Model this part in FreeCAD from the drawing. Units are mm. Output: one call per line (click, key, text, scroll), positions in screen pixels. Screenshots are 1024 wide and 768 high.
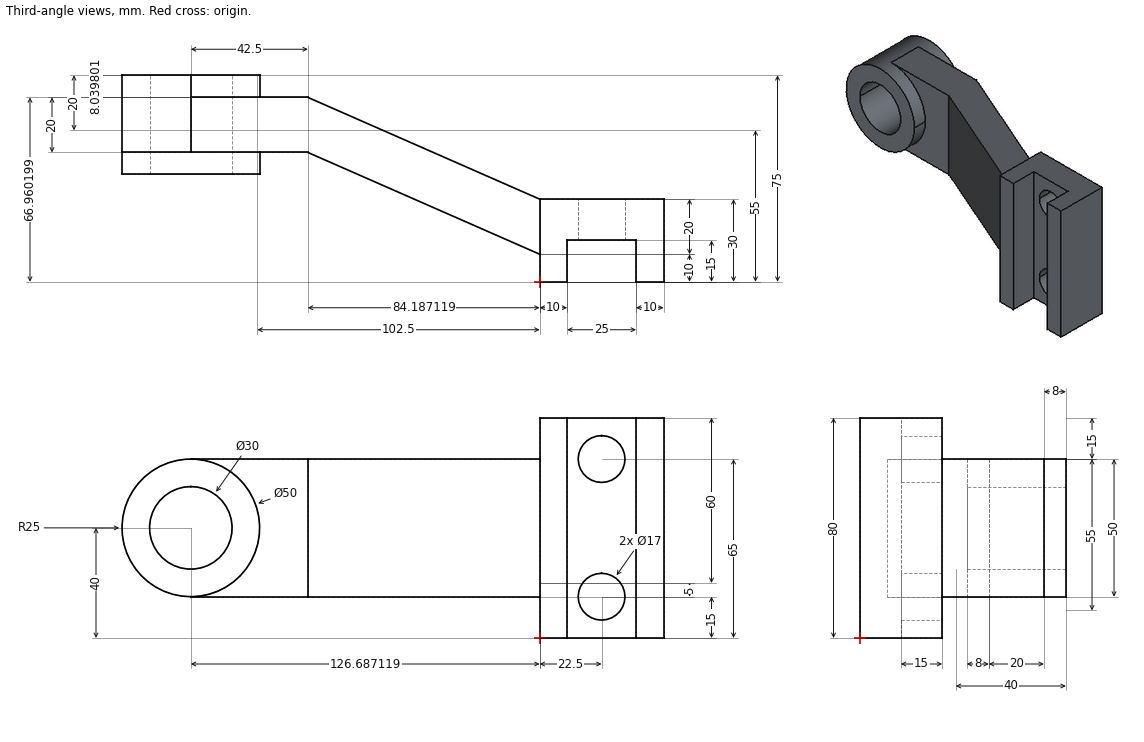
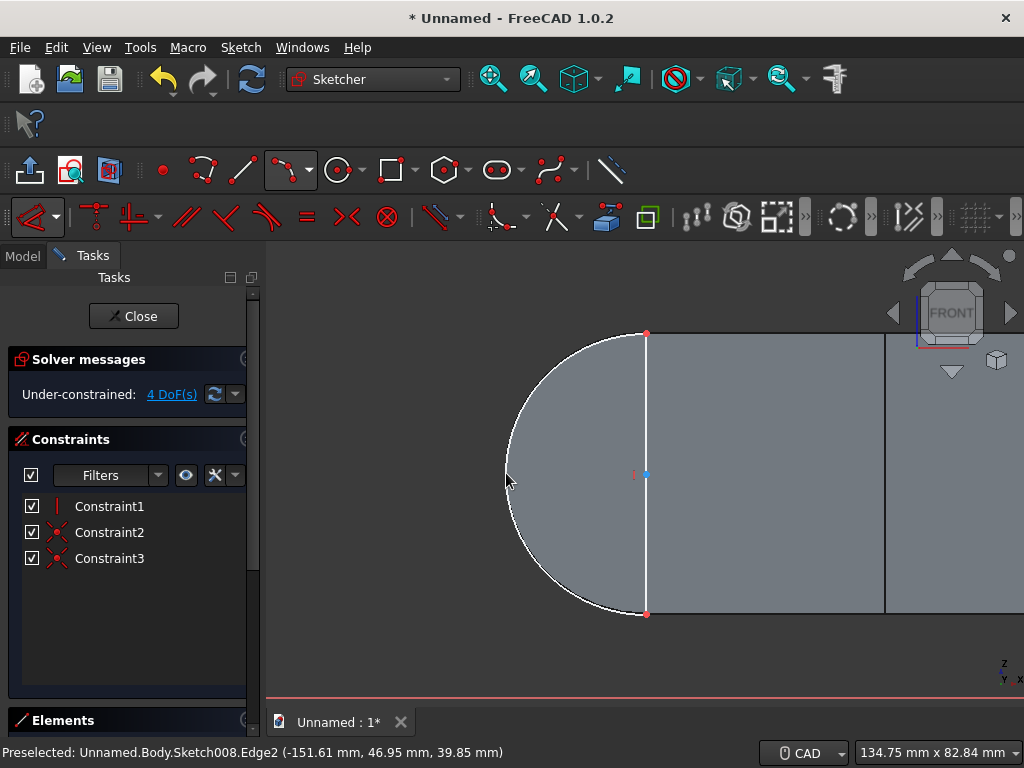
click(533, 392)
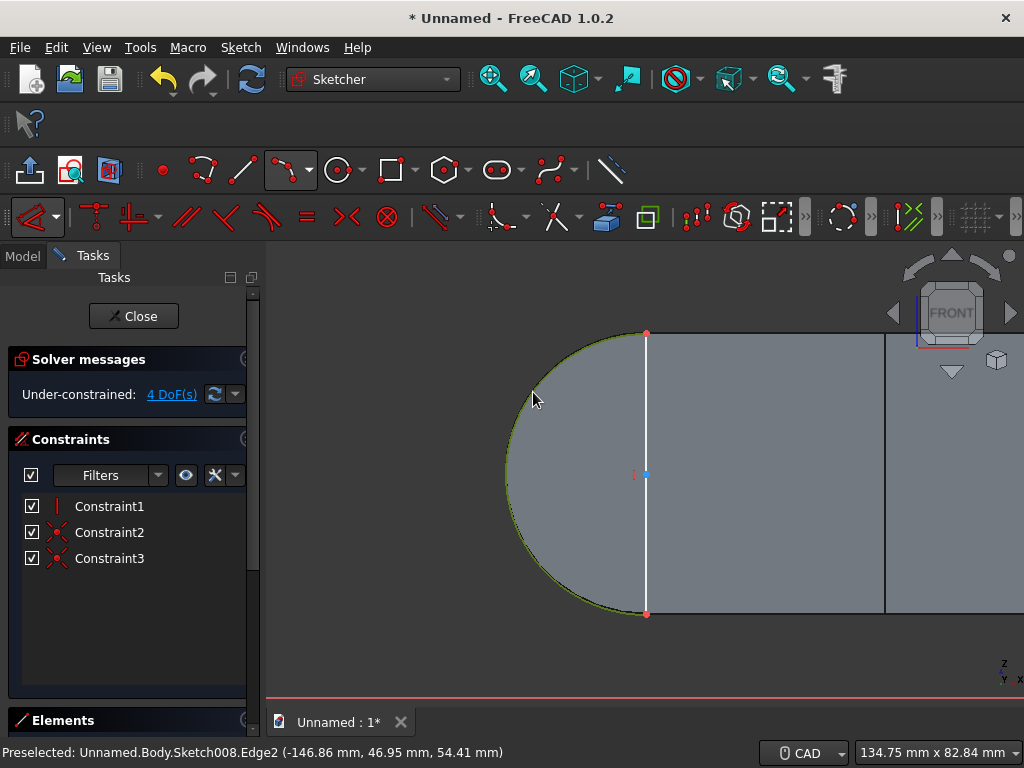
key(k)
key(r)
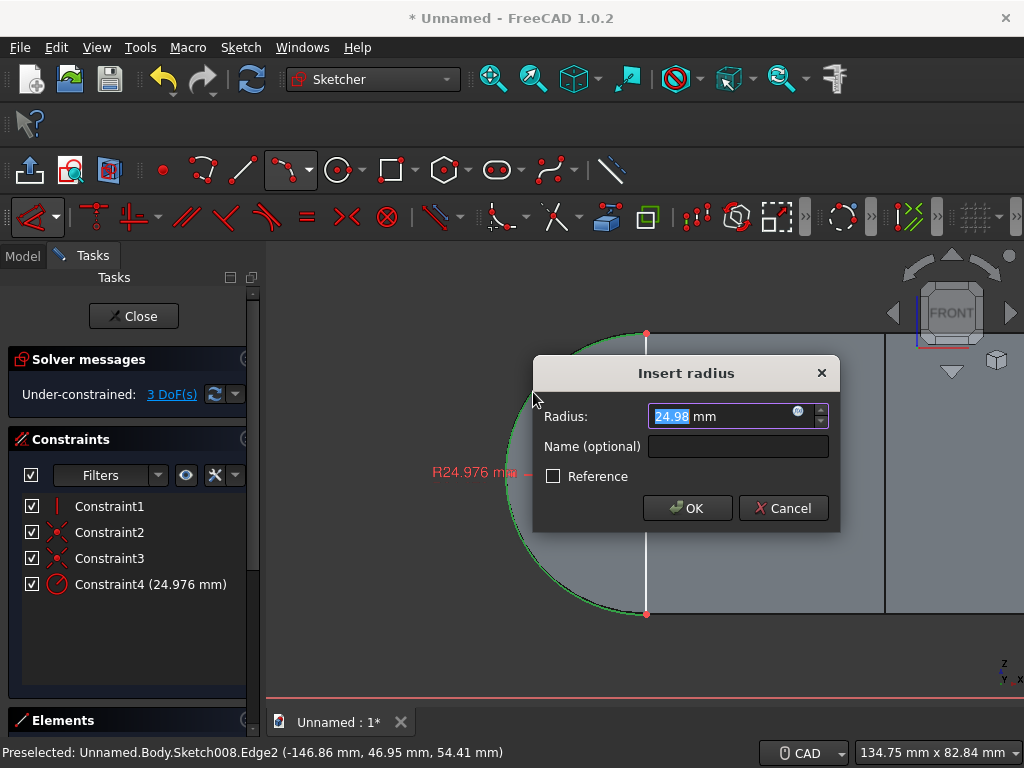
text(25)
key(Return)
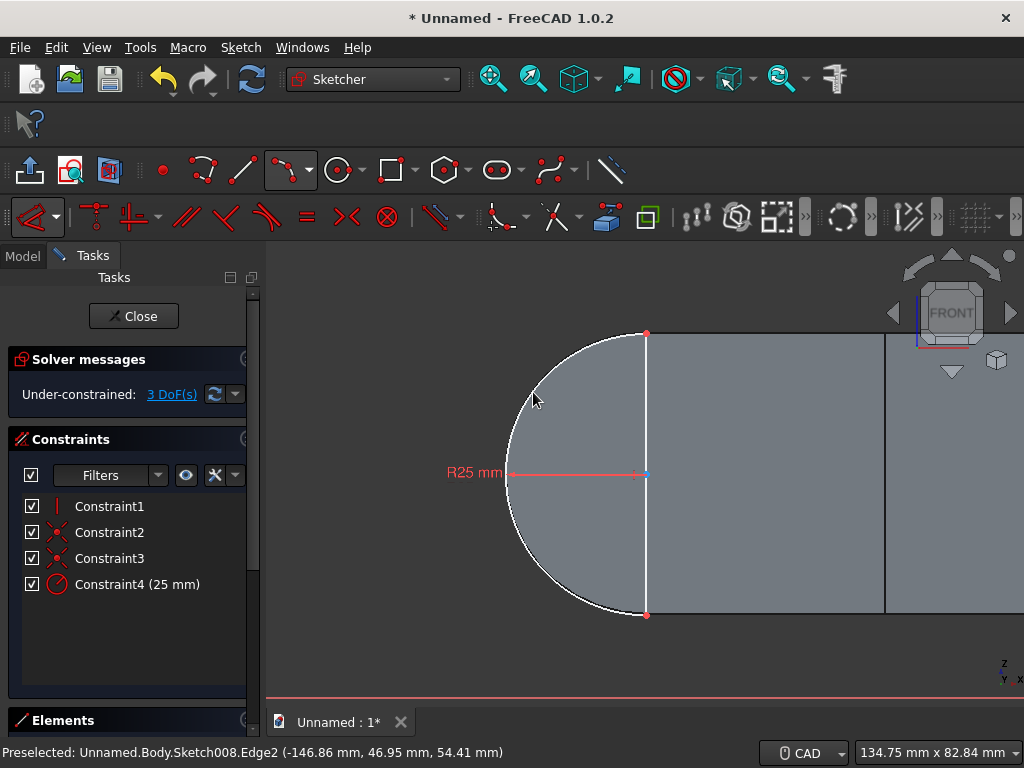
click(646, 615)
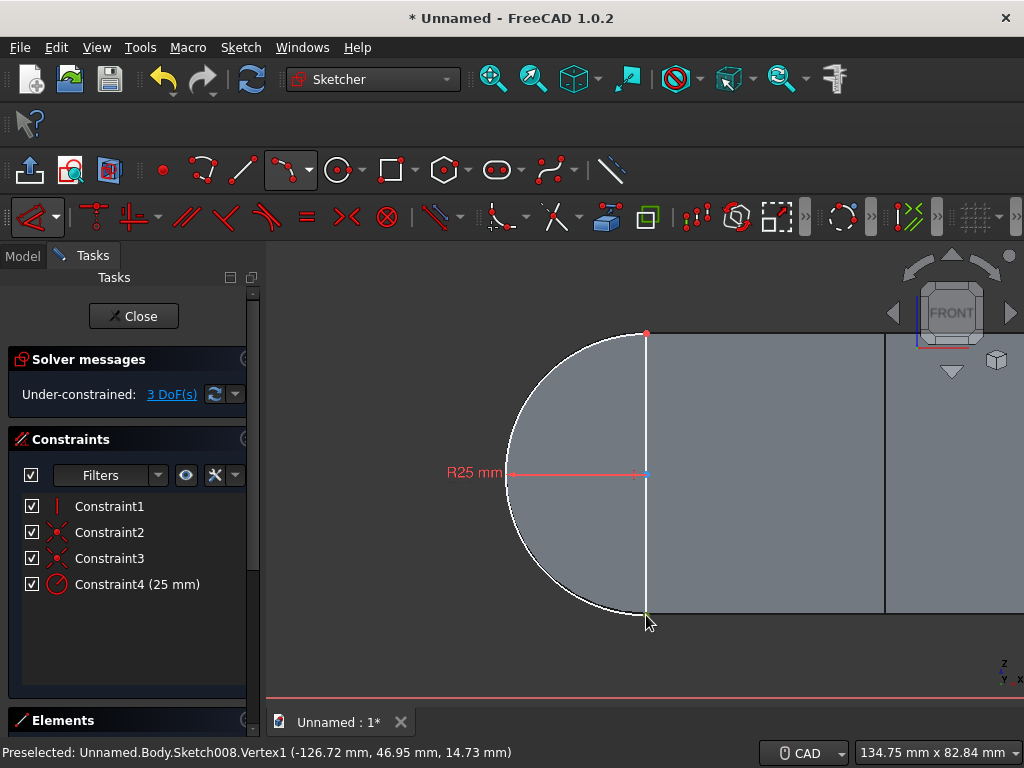
key(i)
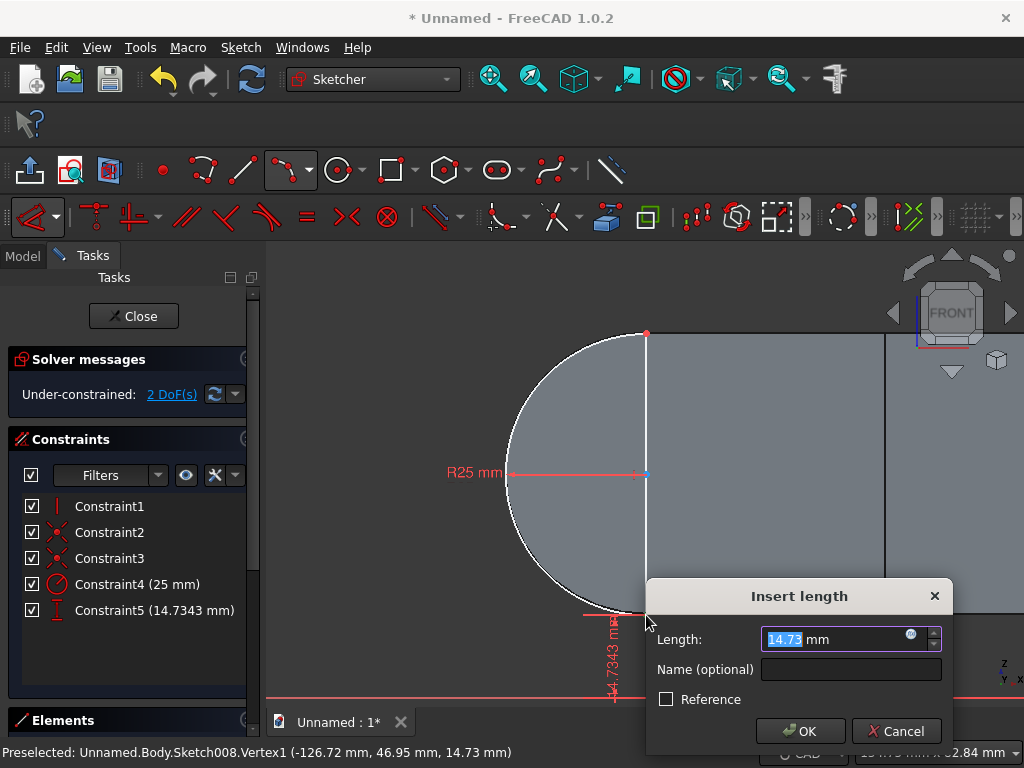
text(15)
key(Return)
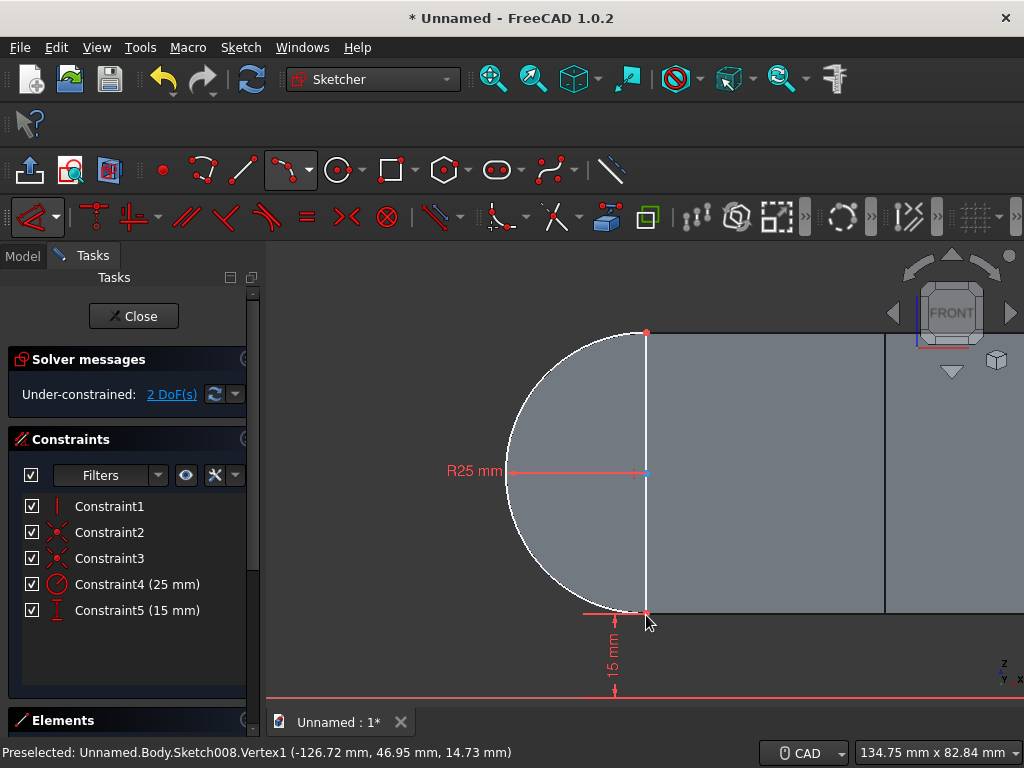
click(646, 614)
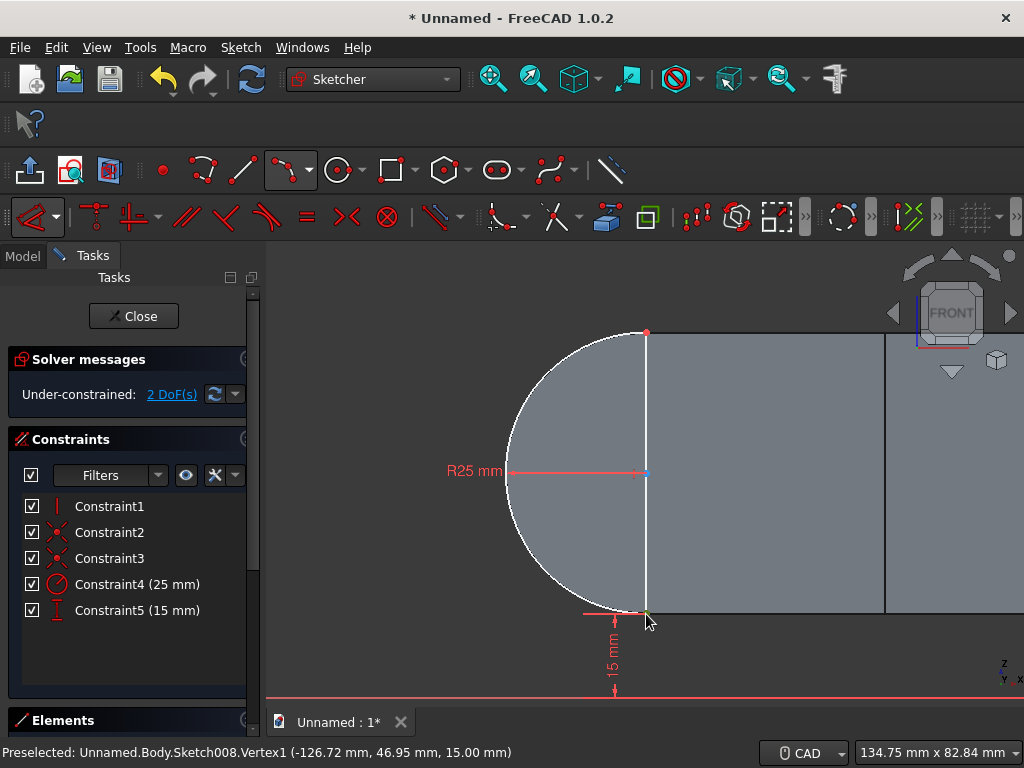
key(l)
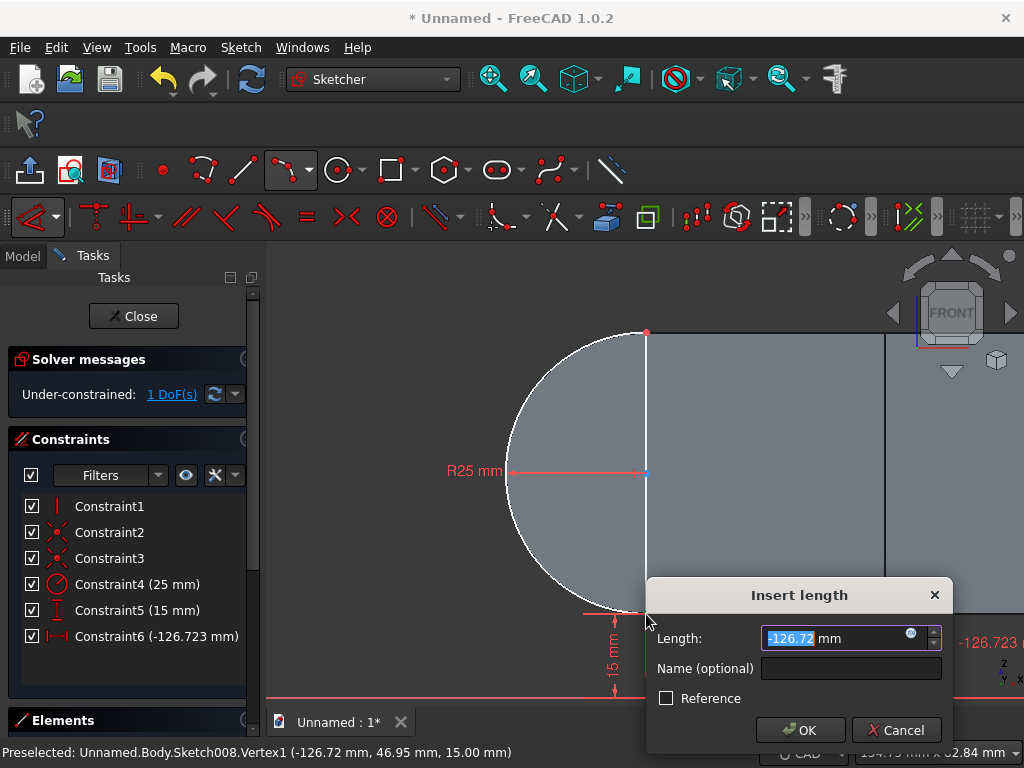
text(-126.687119)
key(Return)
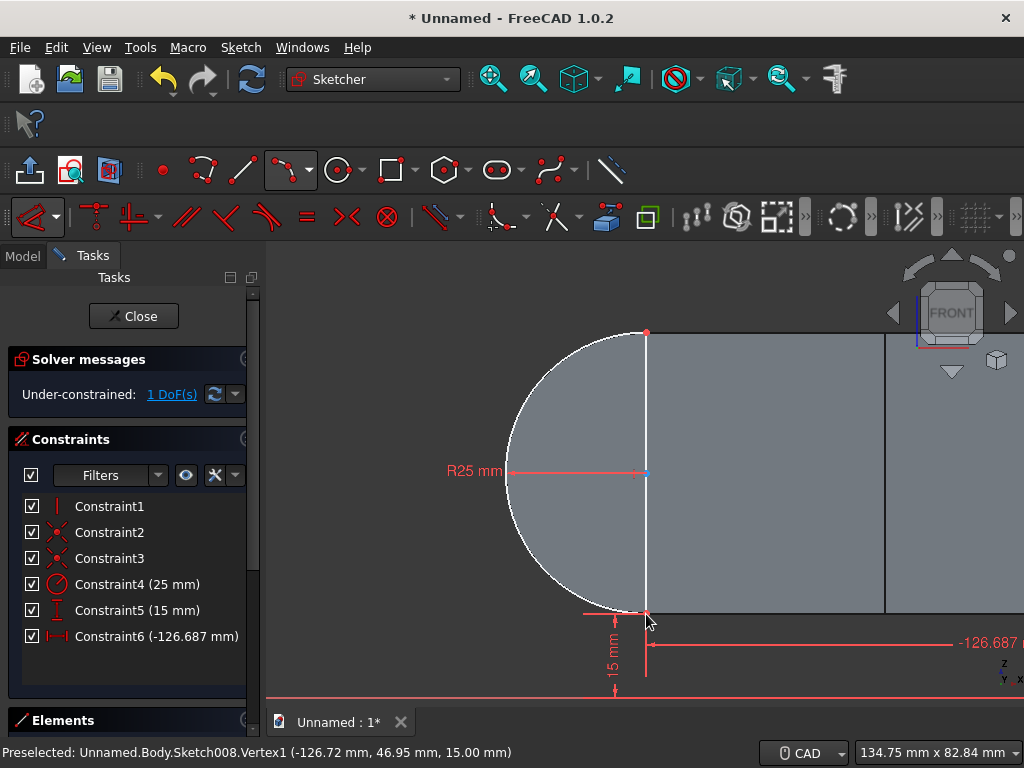
click(647, 473)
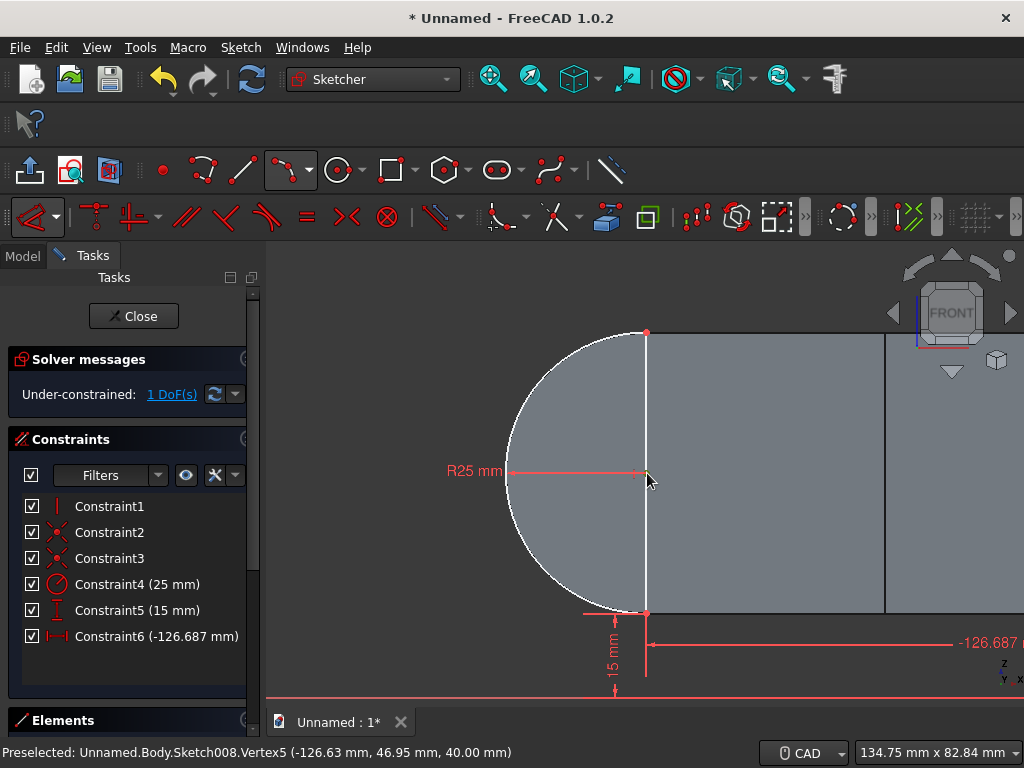
key(l)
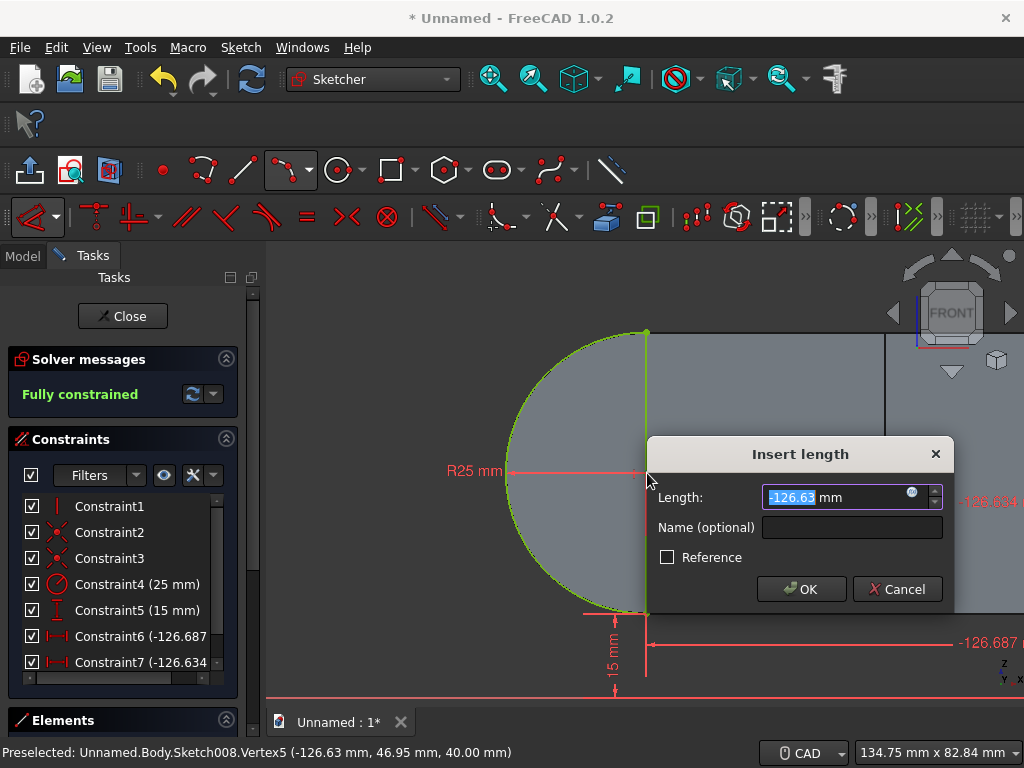
text(-126.687119)
key(Return)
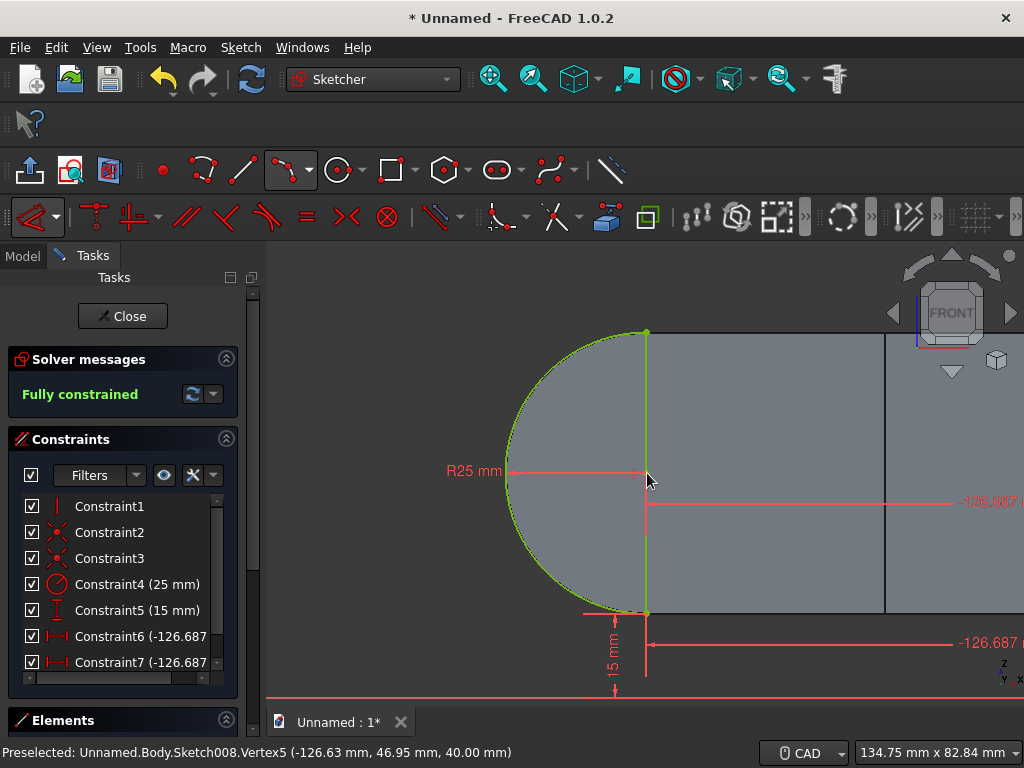
click(123, 316)